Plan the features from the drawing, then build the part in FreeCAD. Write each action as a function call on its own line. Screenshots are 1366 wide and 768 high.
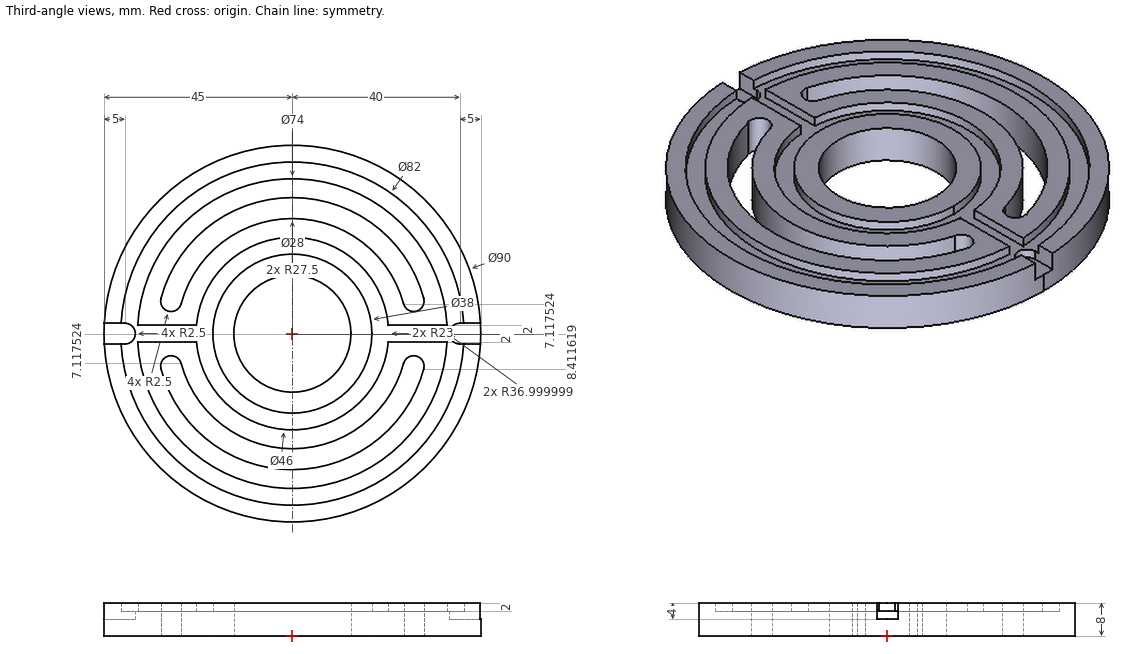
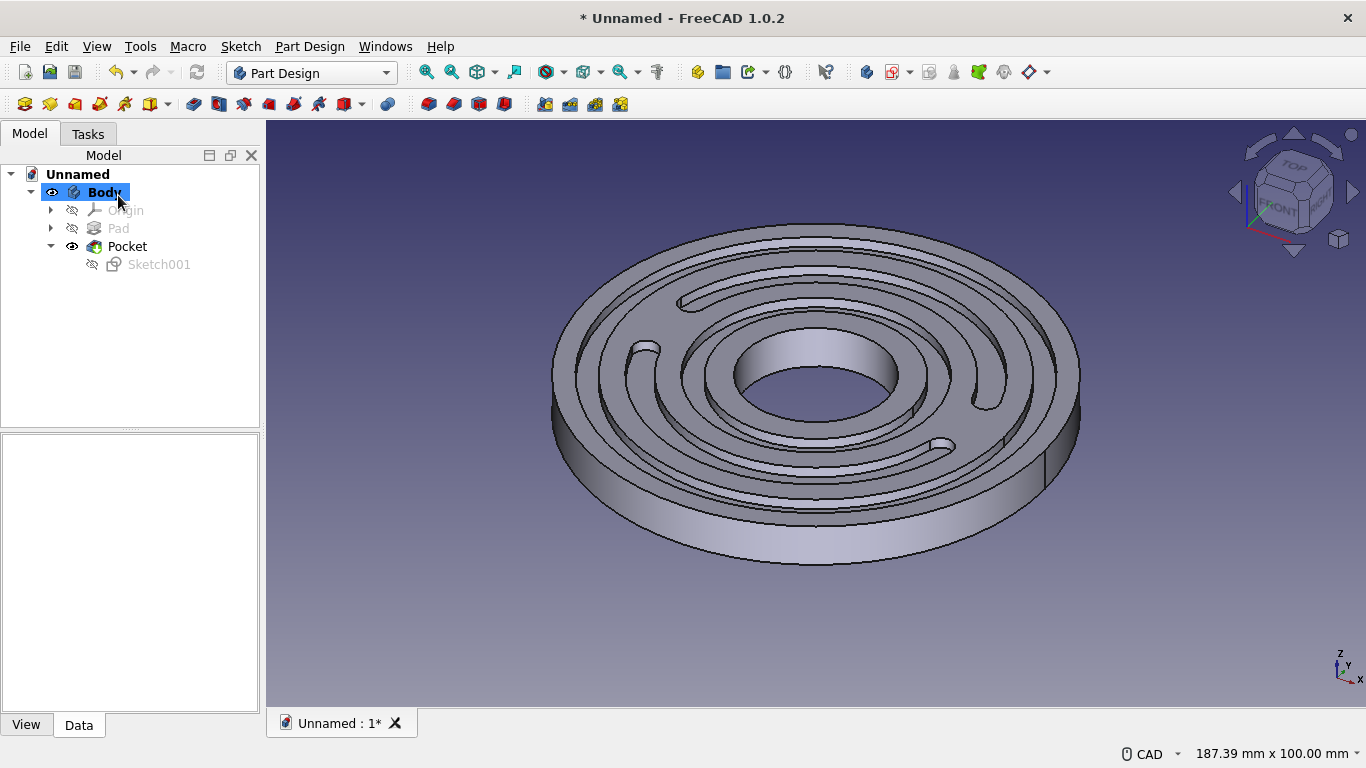
scroll(772, 506, up, 15)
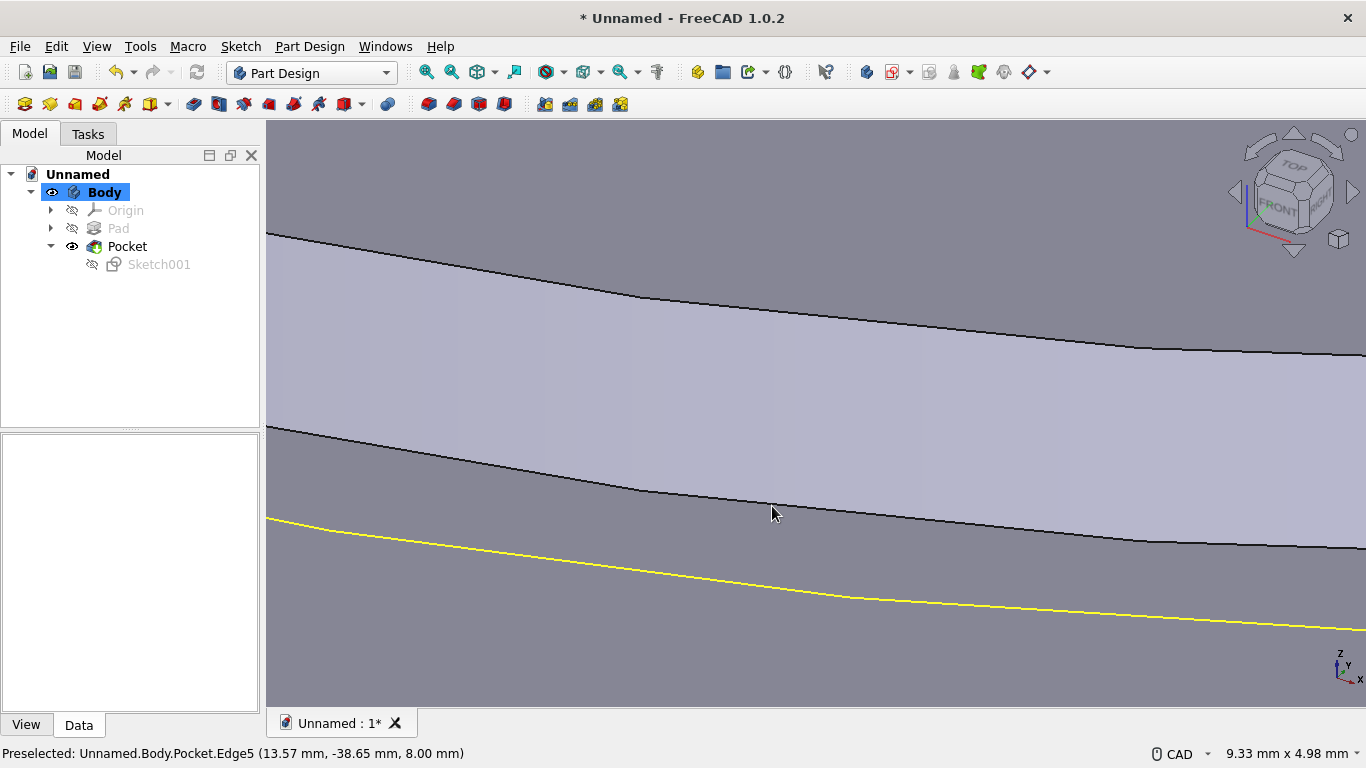
click(771, 509)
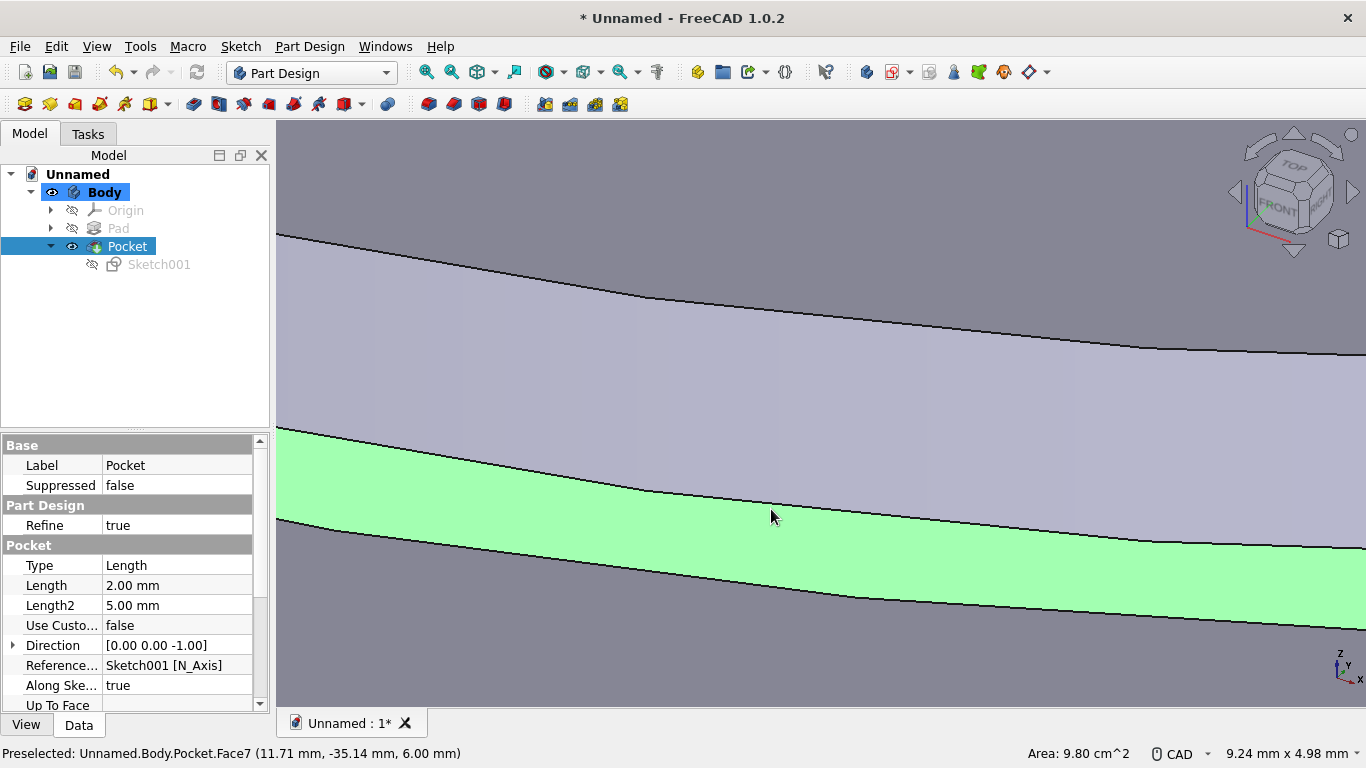
click(892, 72)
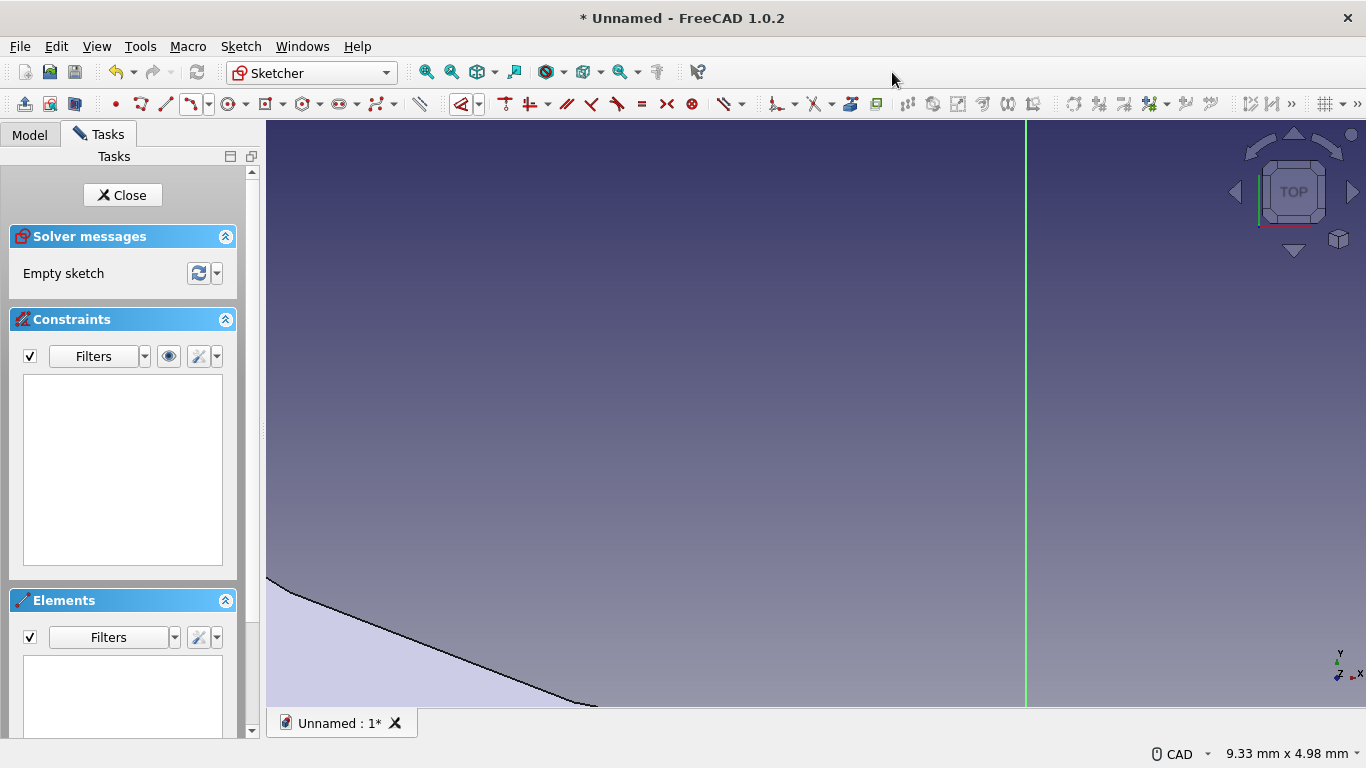
scroll(733, 482, down, 15)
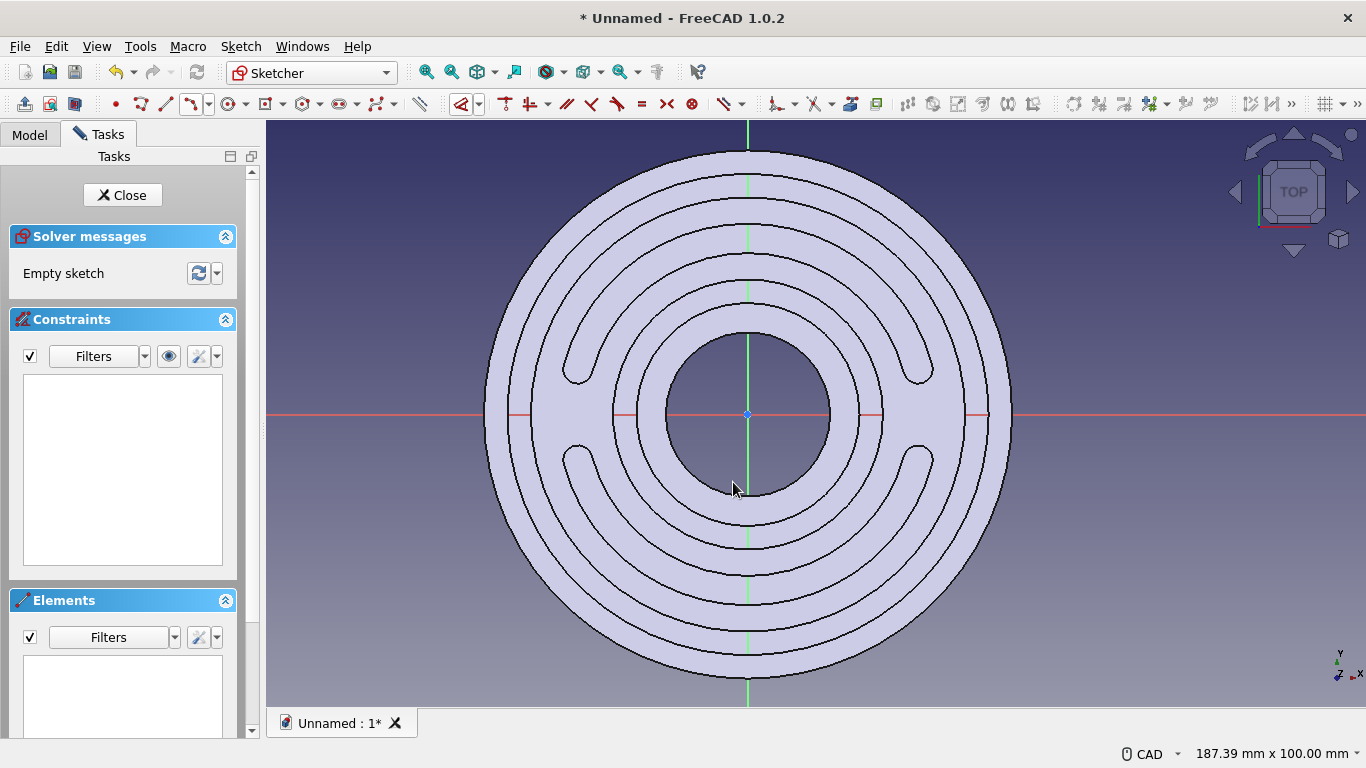
key(g)
key(3)
key(a)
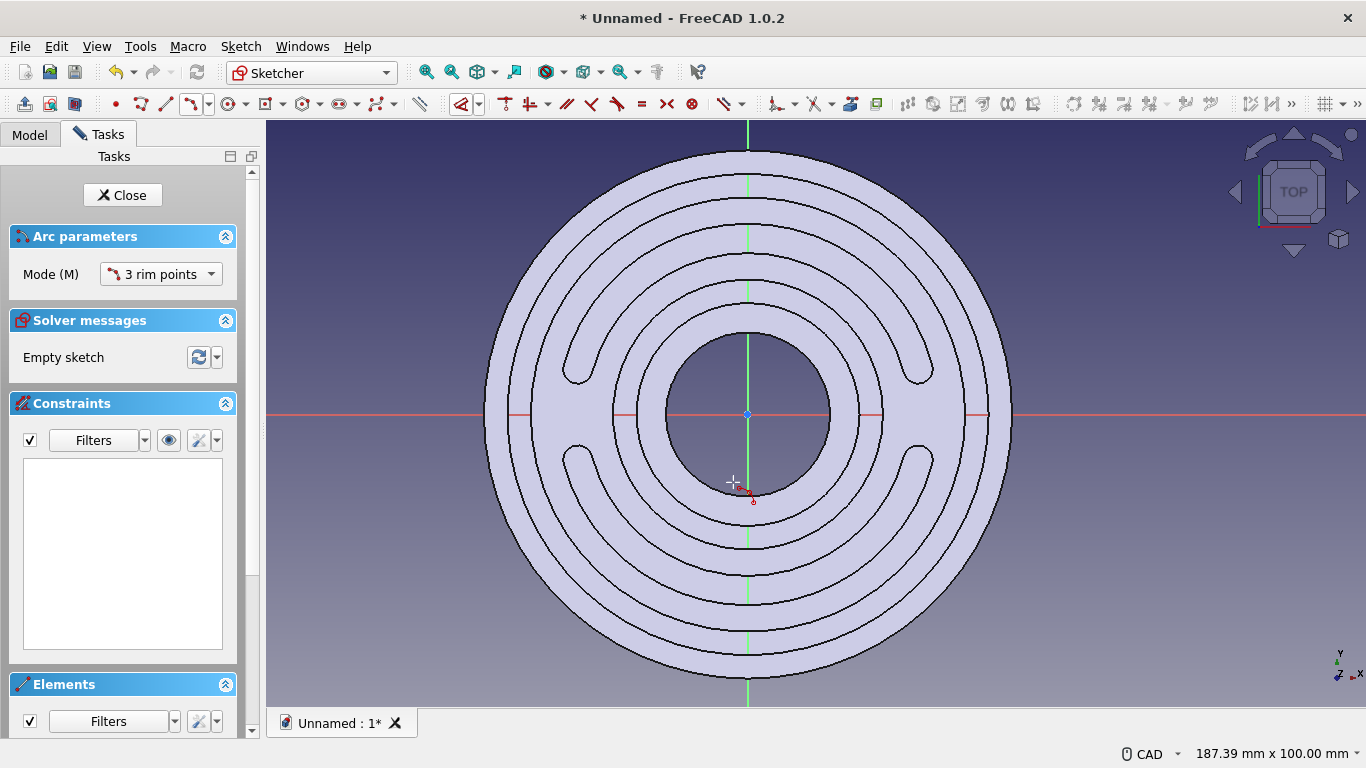
click(592, 373)
click(904, 373)
click(790, 259)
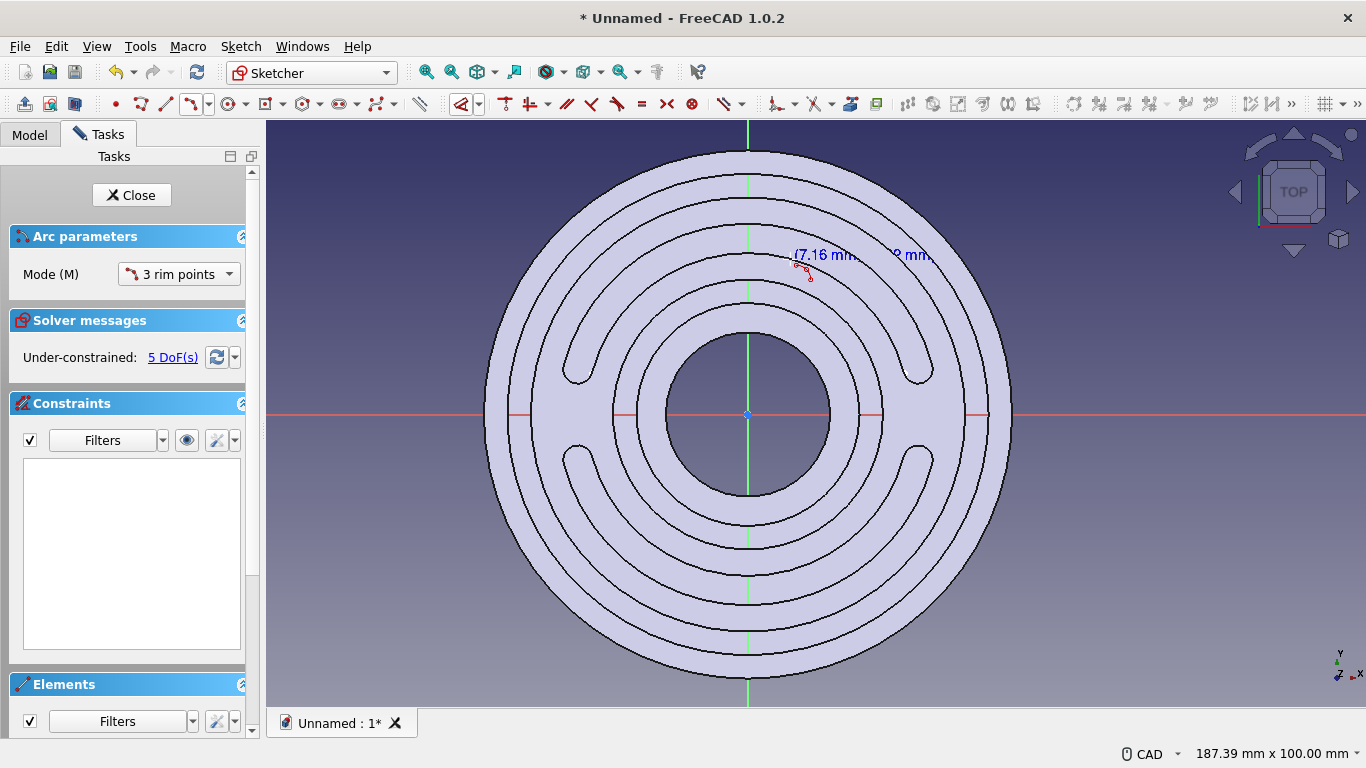
click(904, 374)
click(932, 365)
click(922, 383)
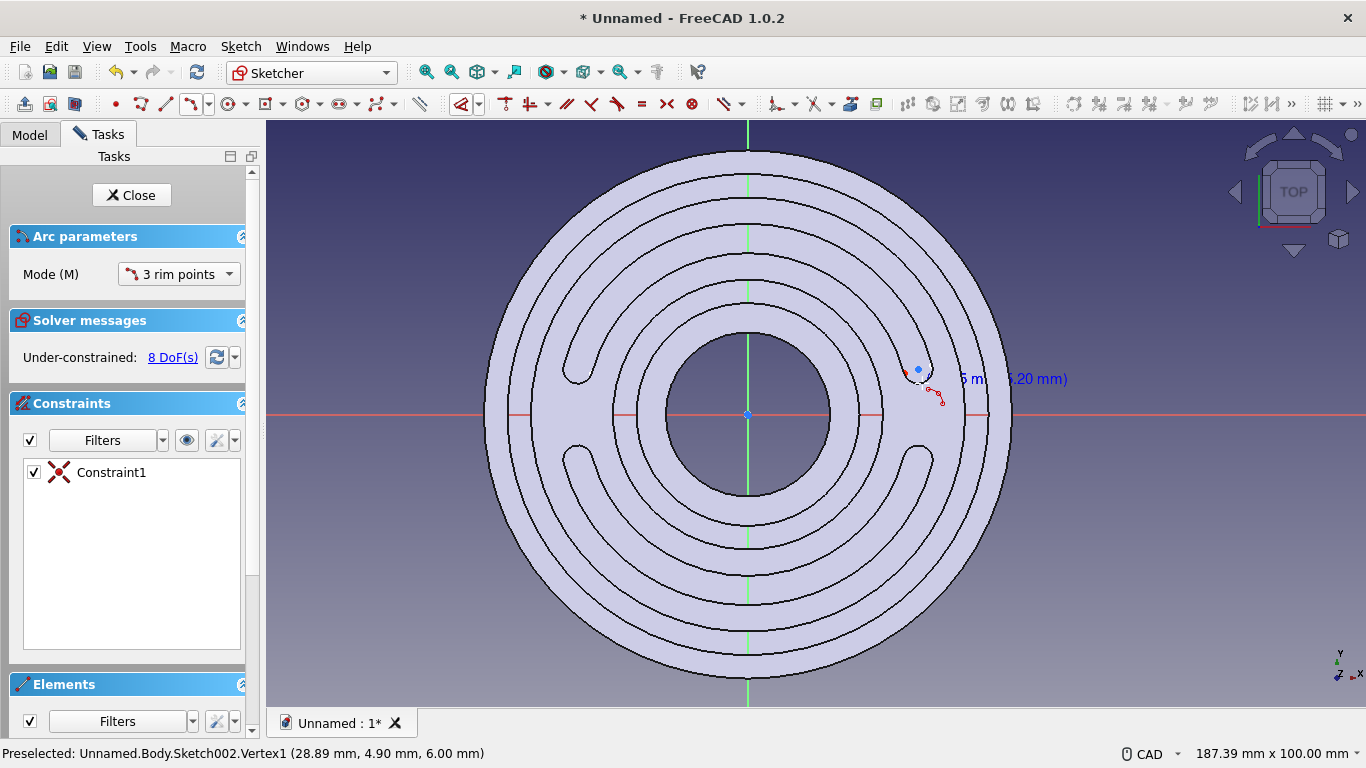
click(932, 366)
click(564, 365)
click(797, 230)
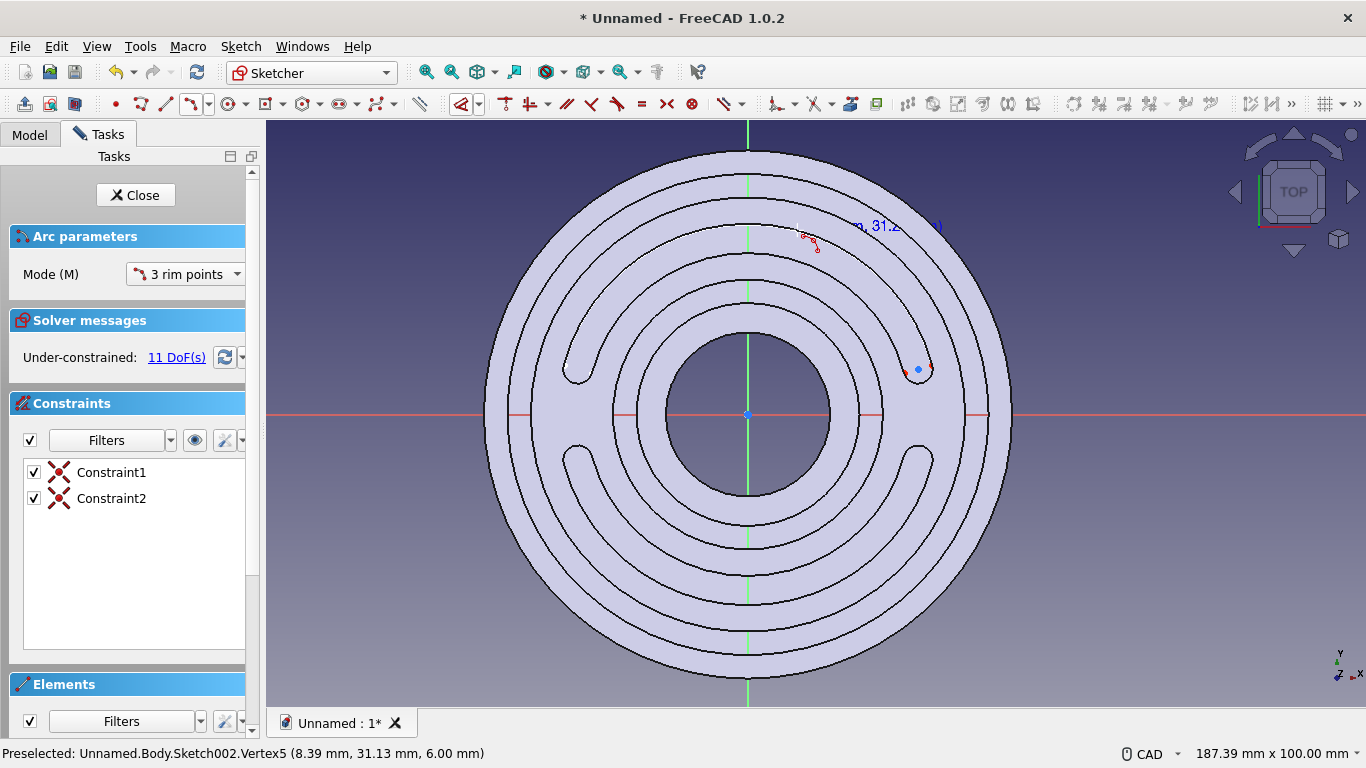
click(564, 366)
click(592, 374)
click(574, 383)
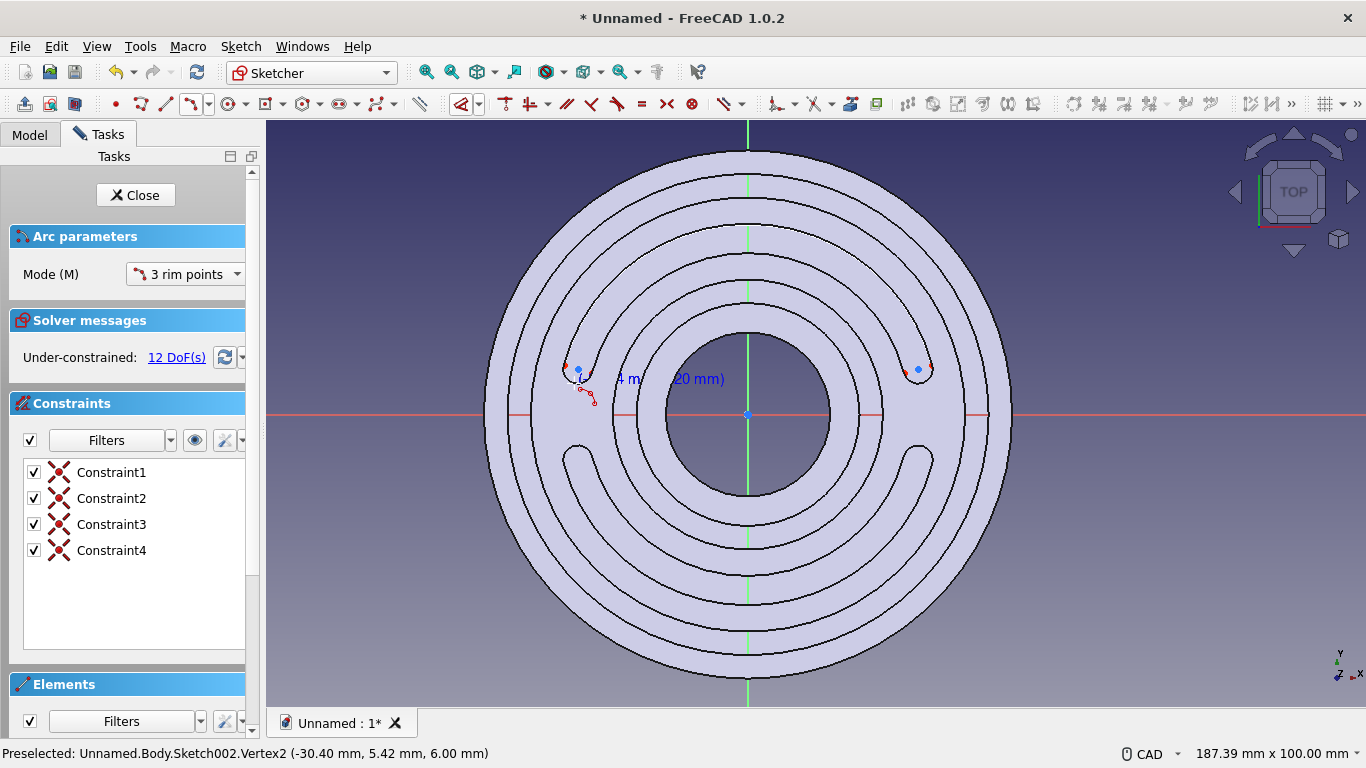
click(592, 456)
click(564, 464)
click(574, 446)